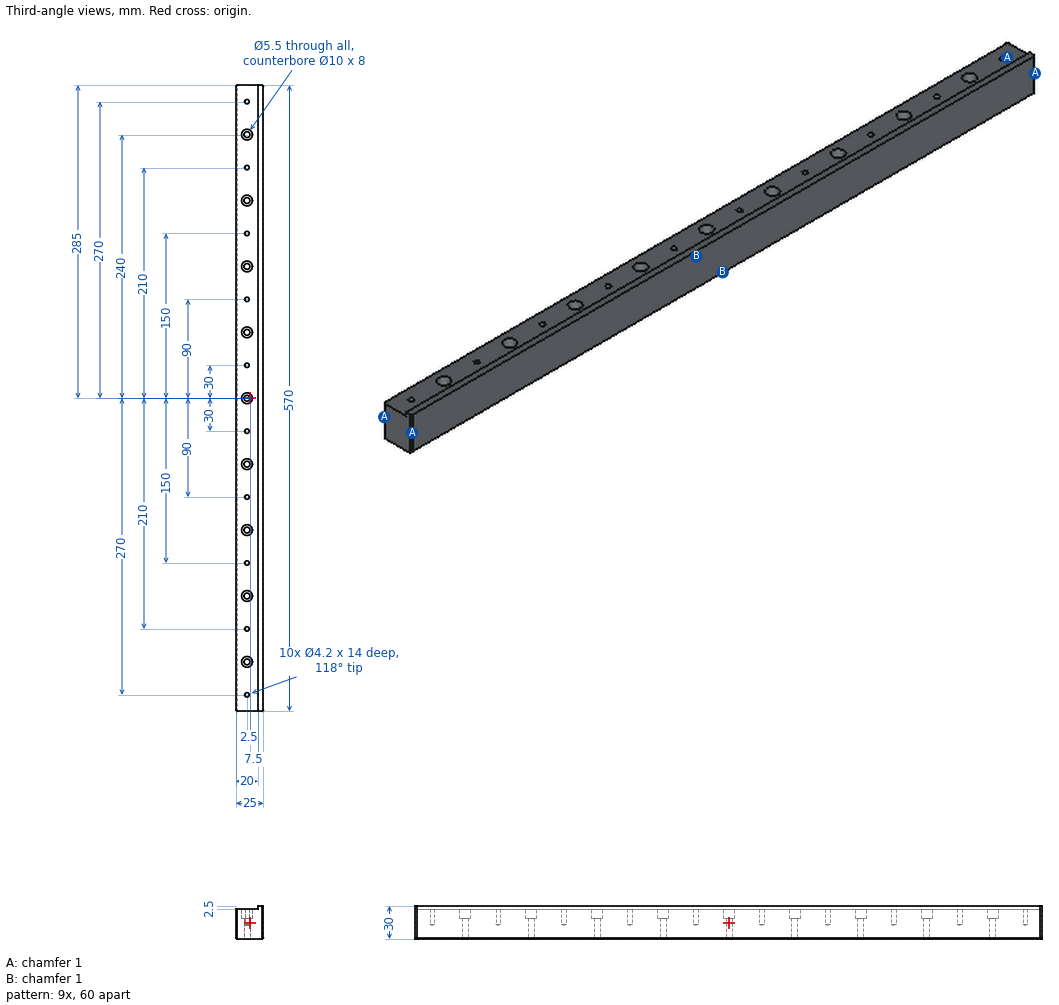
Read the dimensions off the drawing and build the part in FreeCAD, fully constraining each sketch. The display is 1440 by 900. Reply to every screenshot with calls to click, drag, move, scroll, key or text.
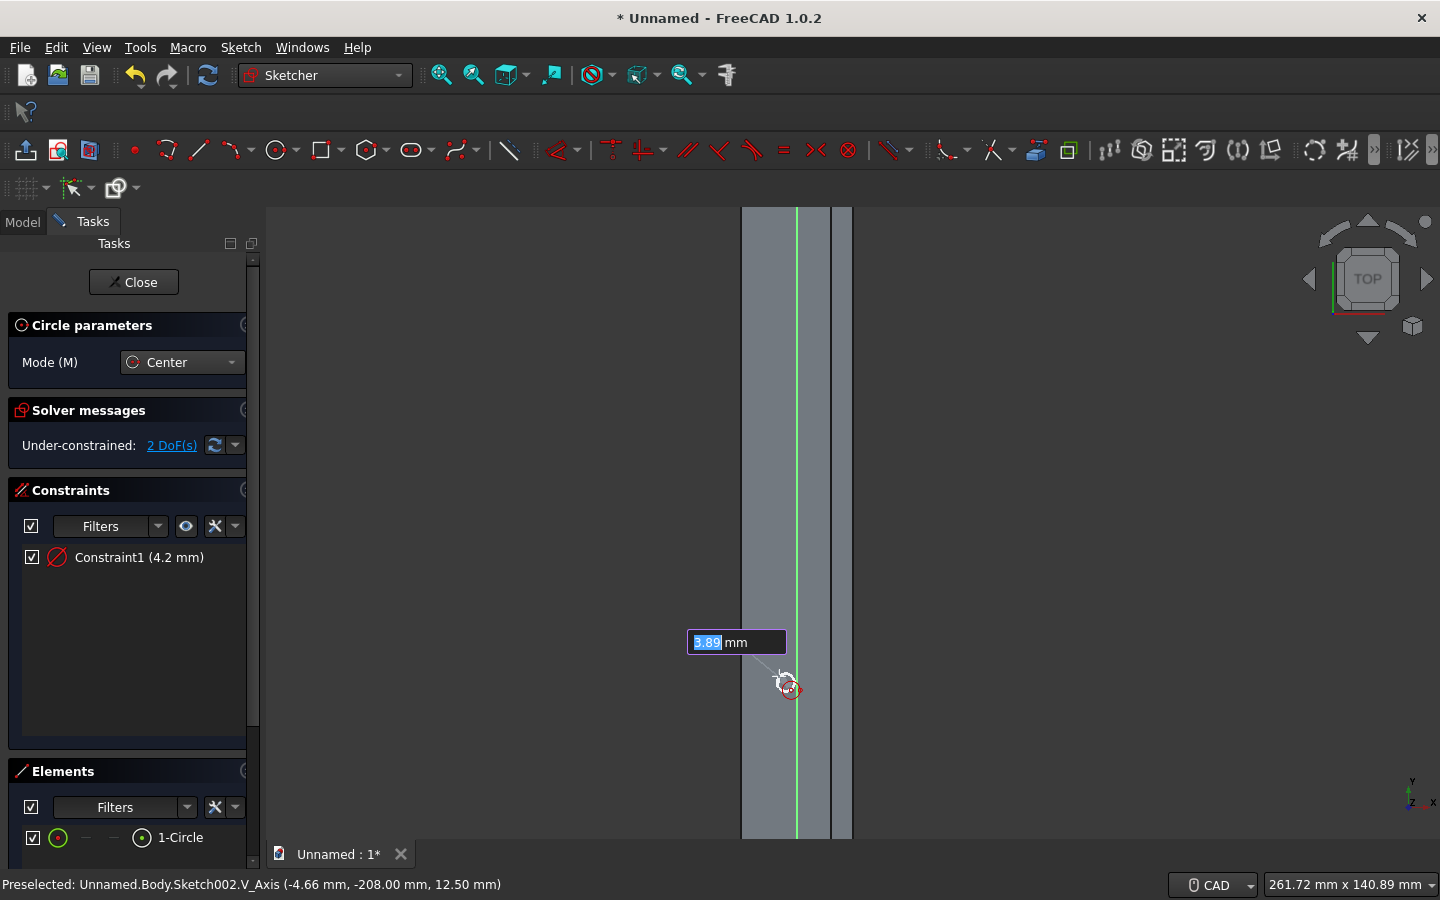
text(4.2)
key(Return)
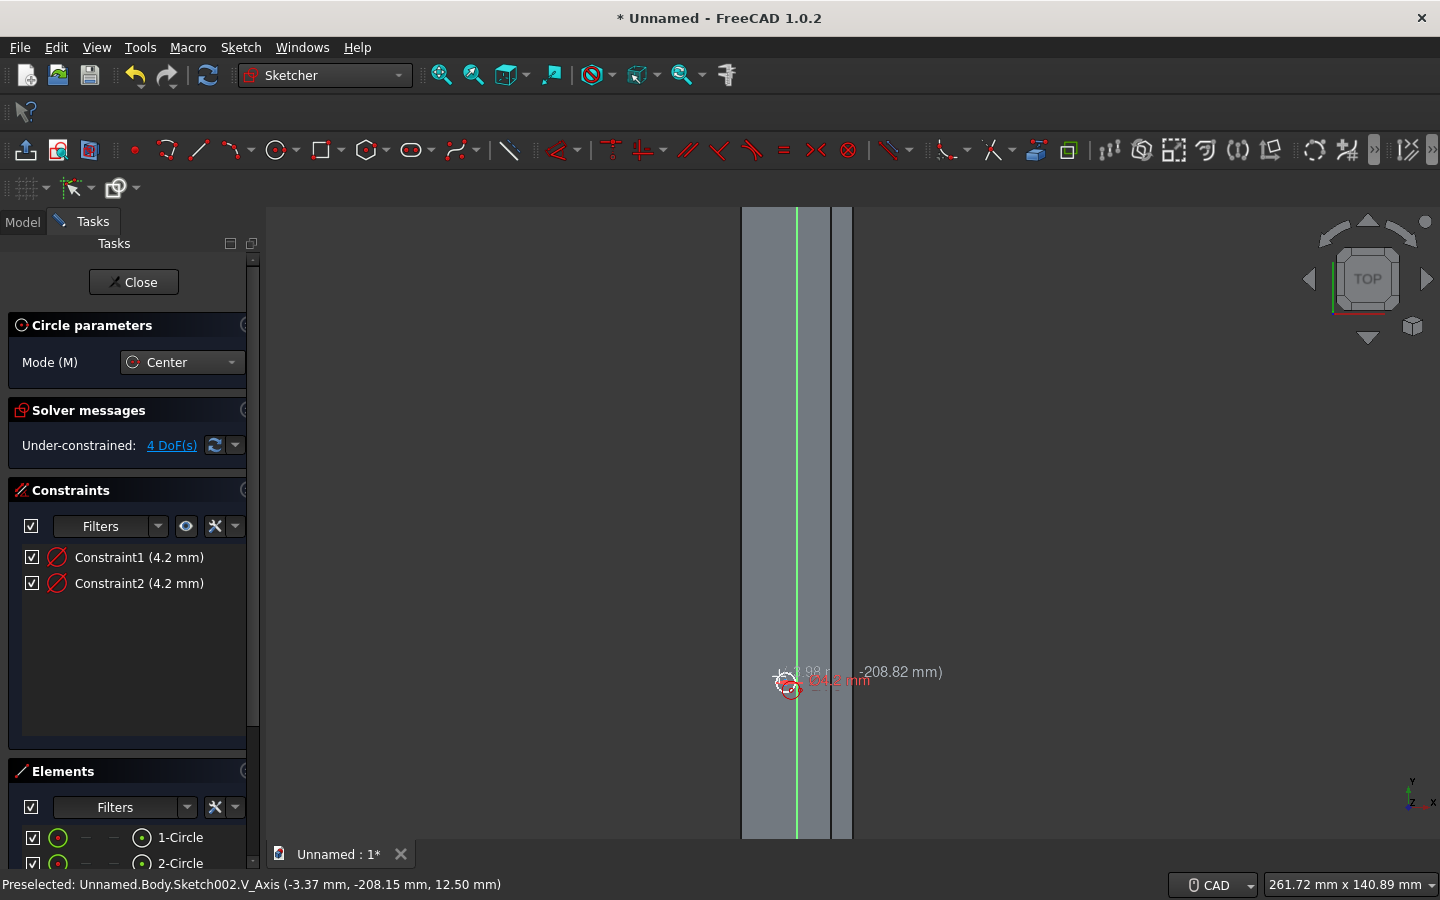
scroll(786, 413, up, 5)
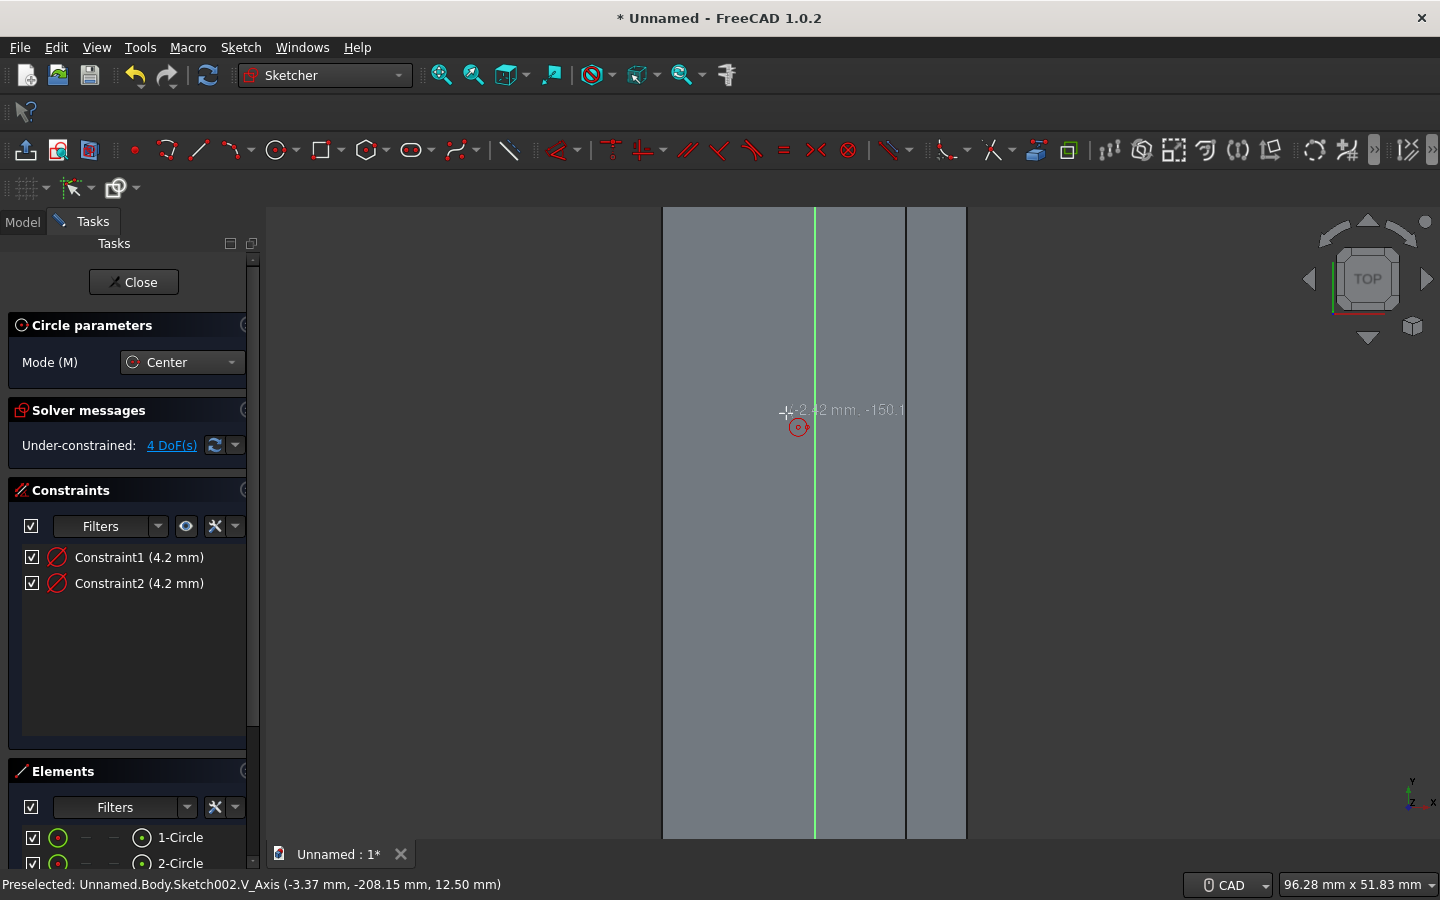
click(784, 413)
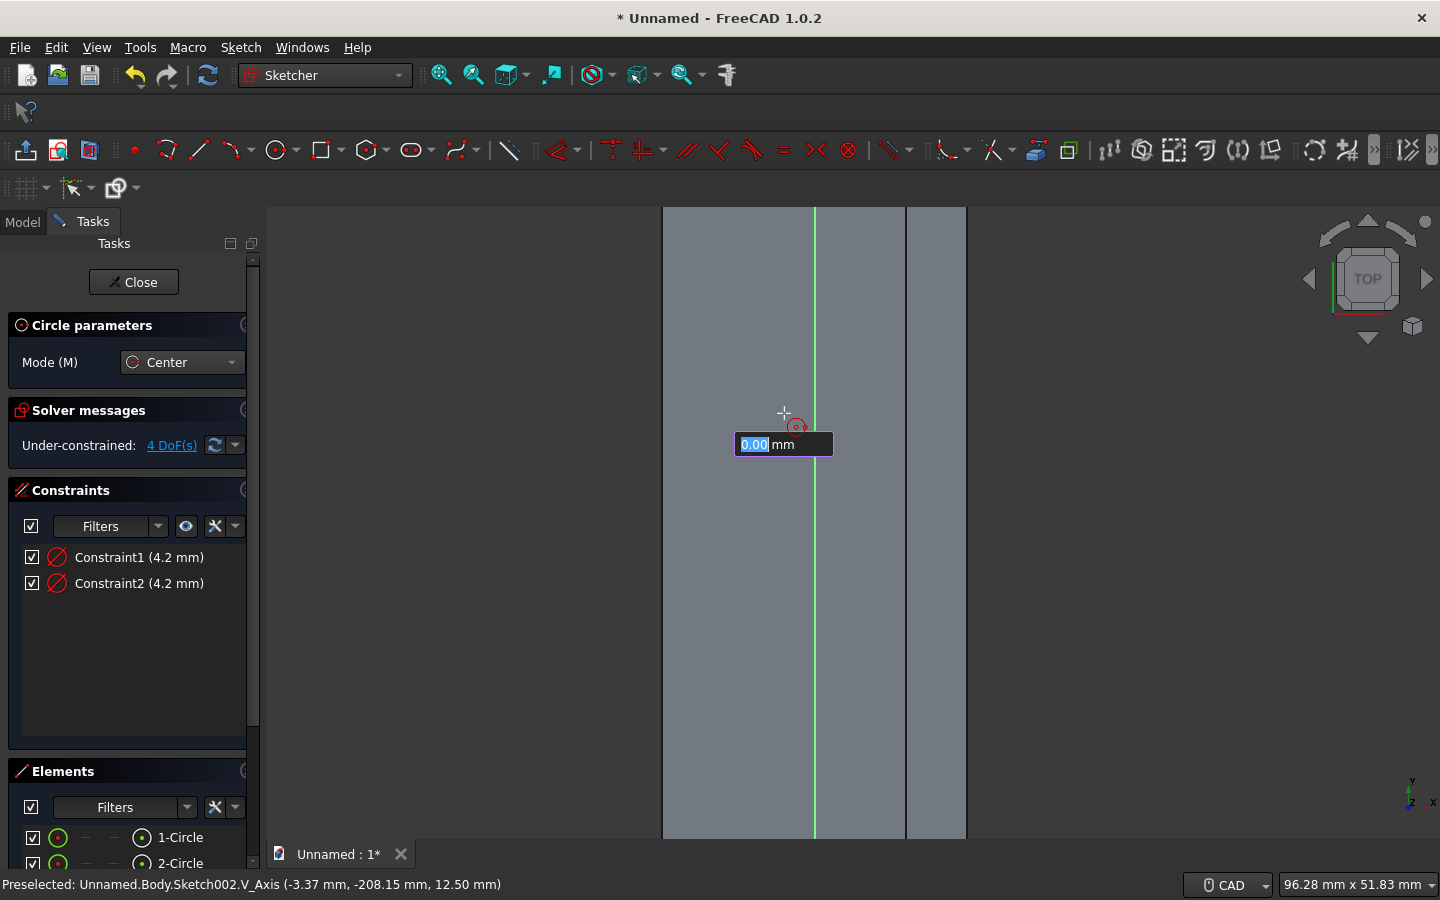
scroll(784, 649, down, 14)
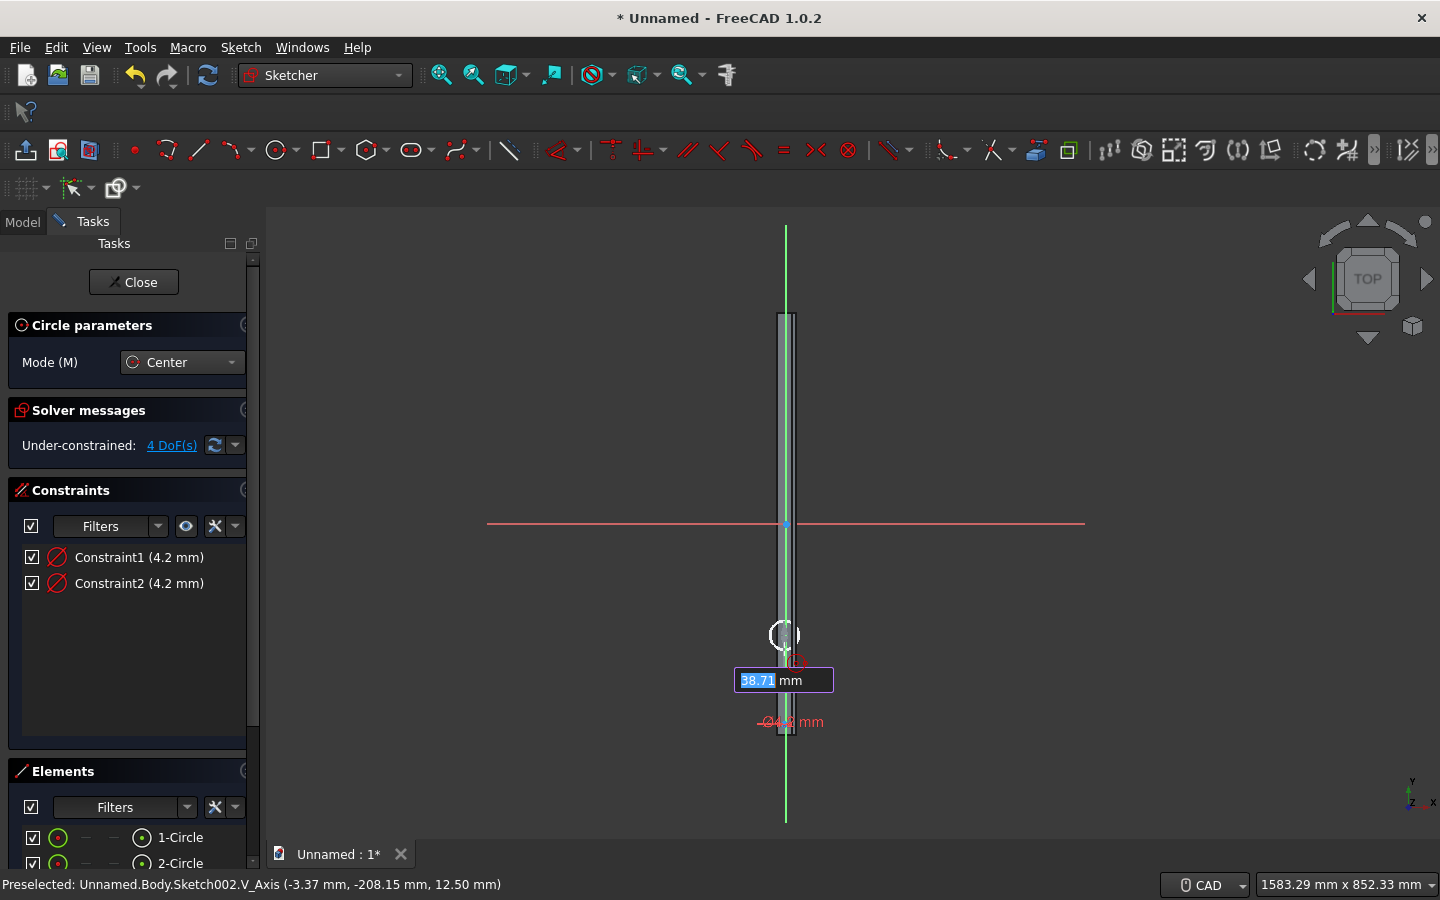
scroll(783, 634, up, 9)
move(783, 632)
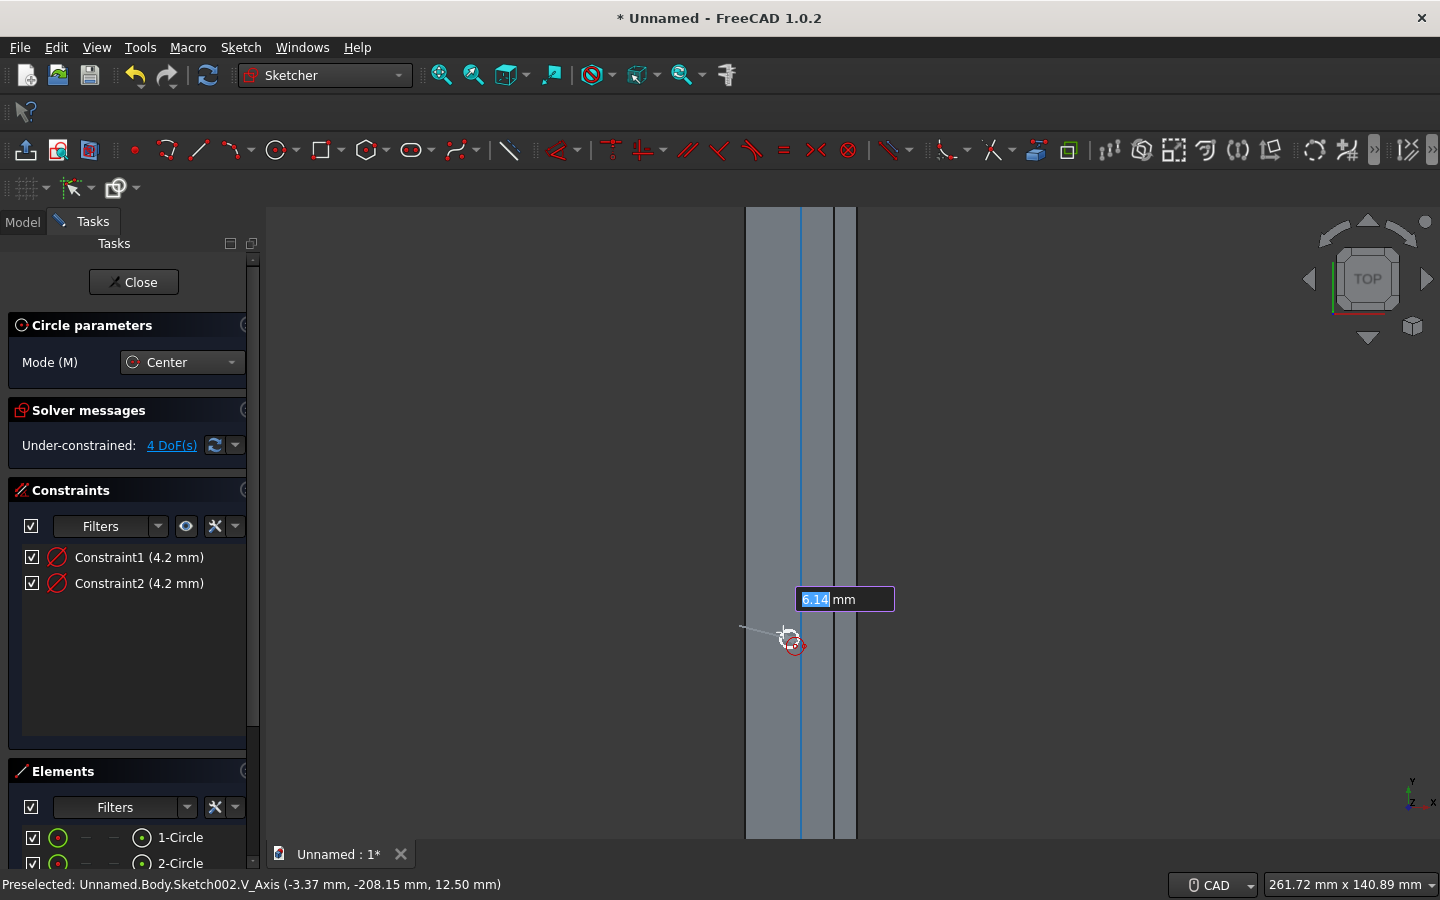
text(4.2)
key(Return)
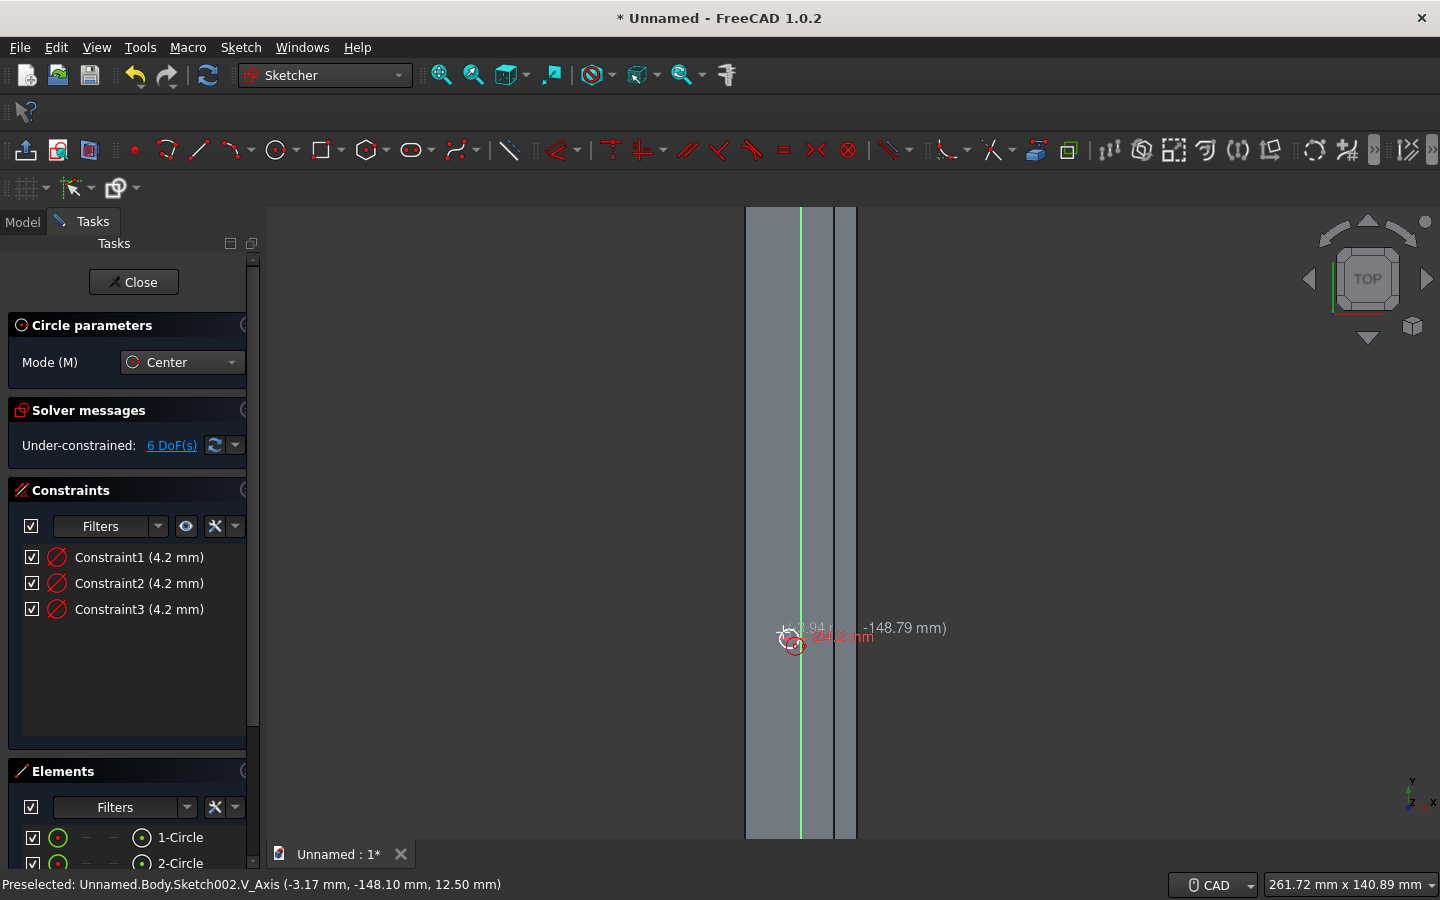
scroll(789, 369, up, 5)